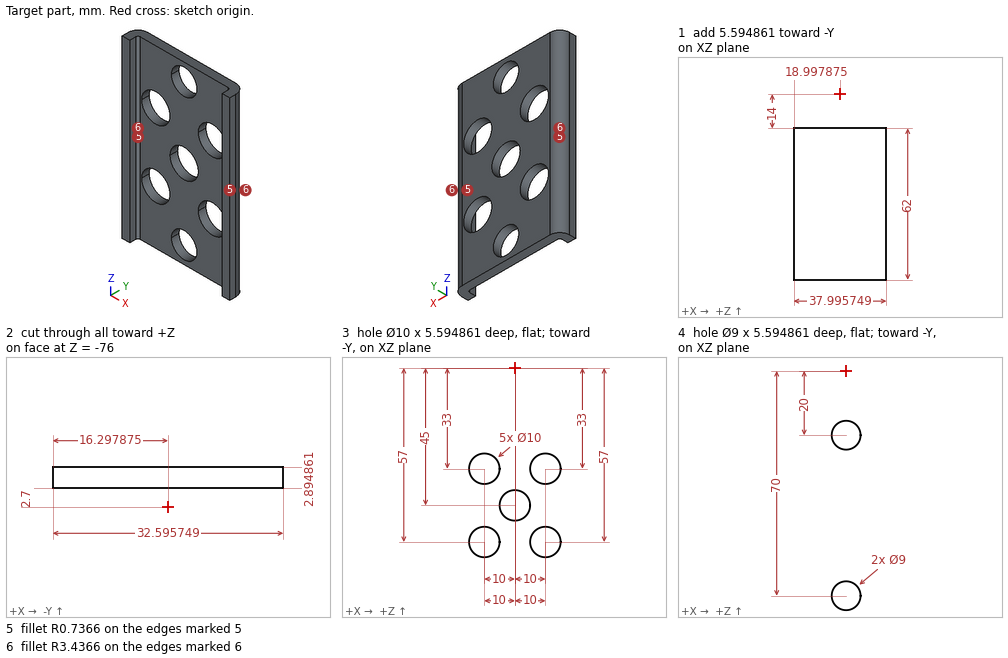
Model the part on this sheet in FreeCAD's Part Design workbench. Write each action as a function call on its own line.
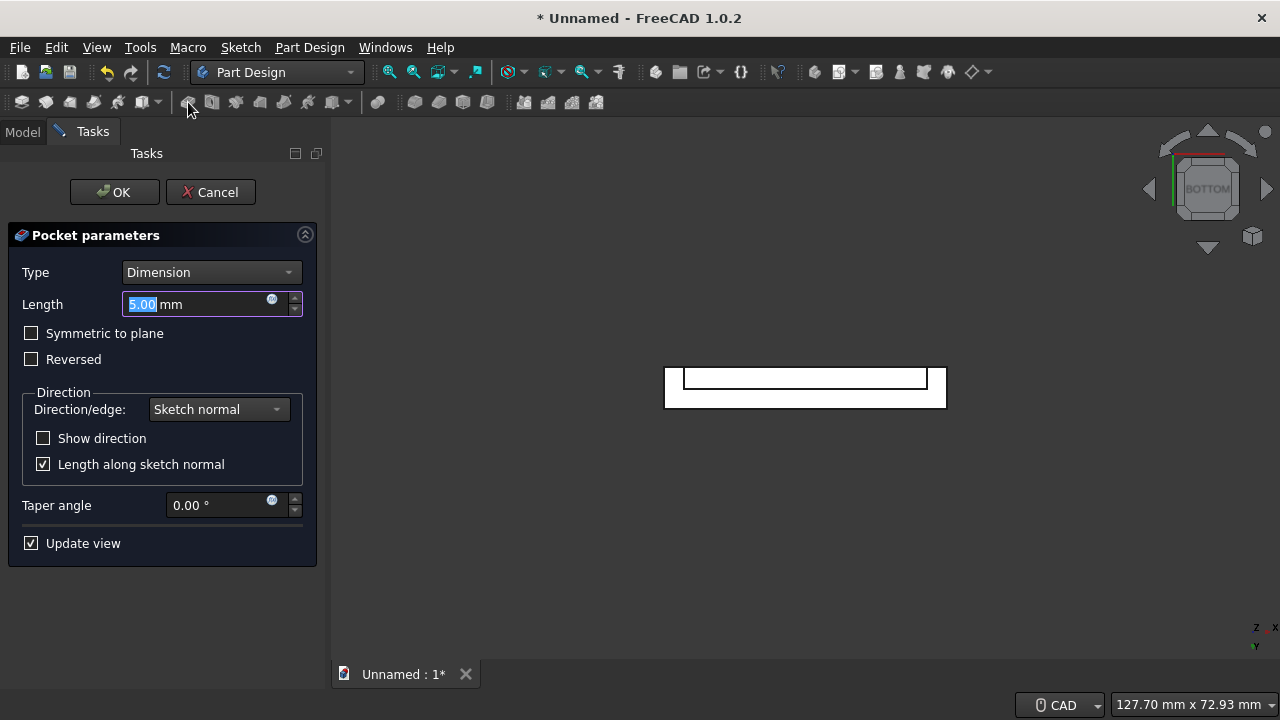
click(212, 272)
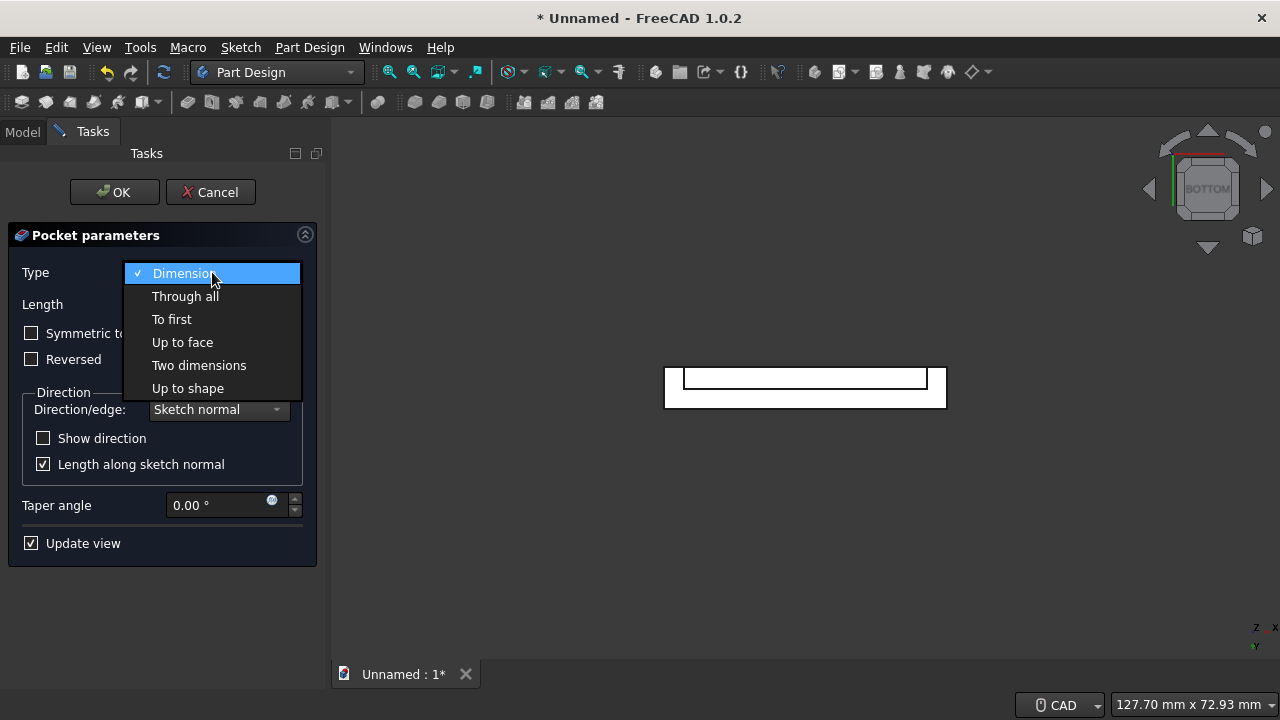
click(212, 296)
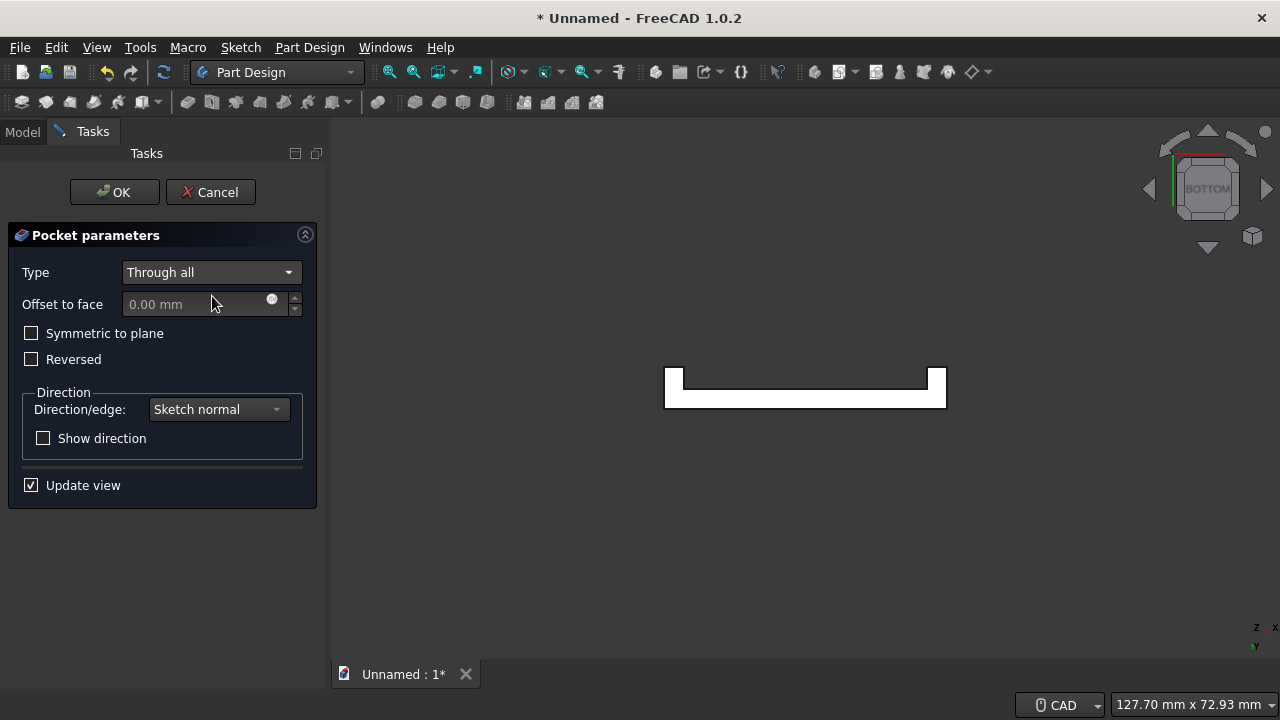
click(115, 192)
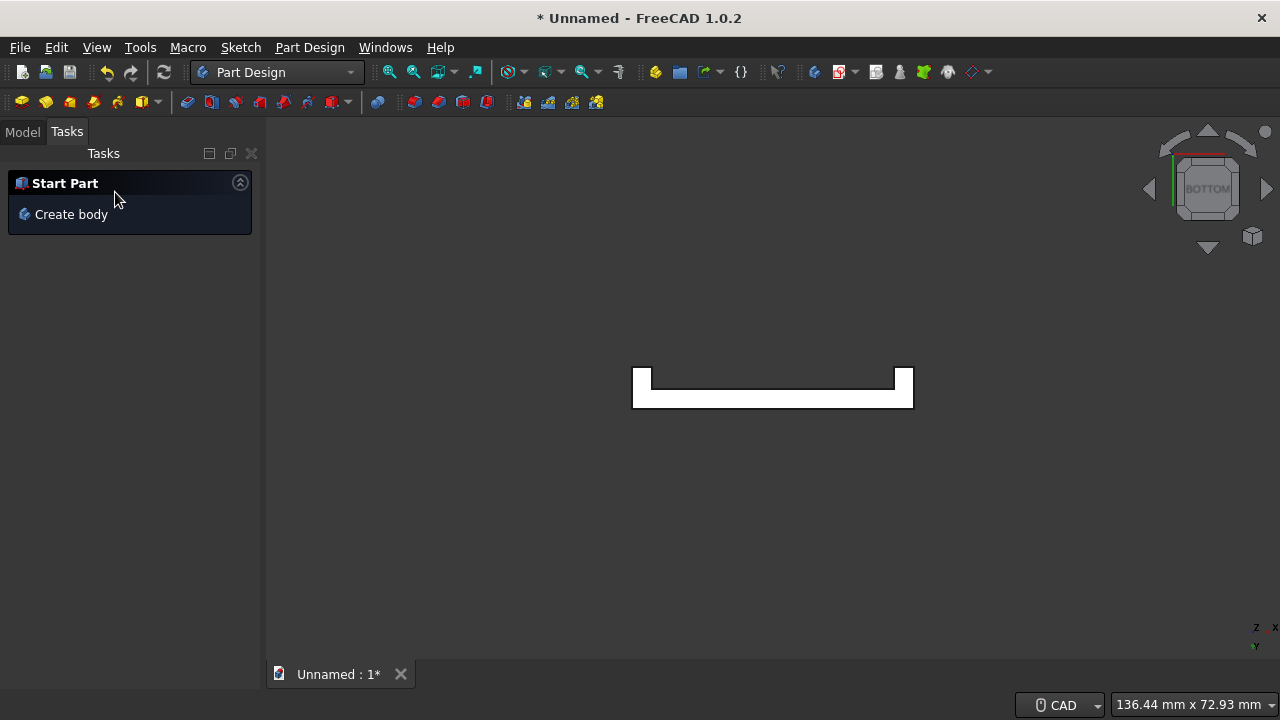
key(v)
key(f)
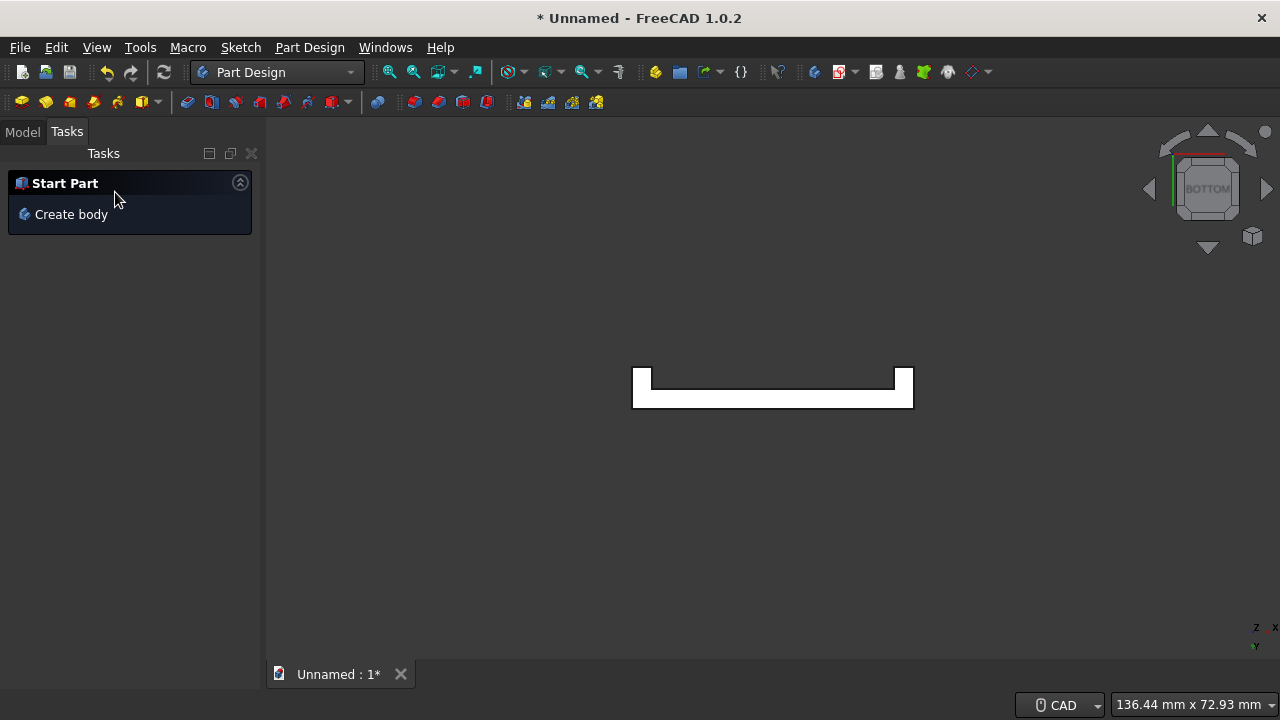
click(840, 72)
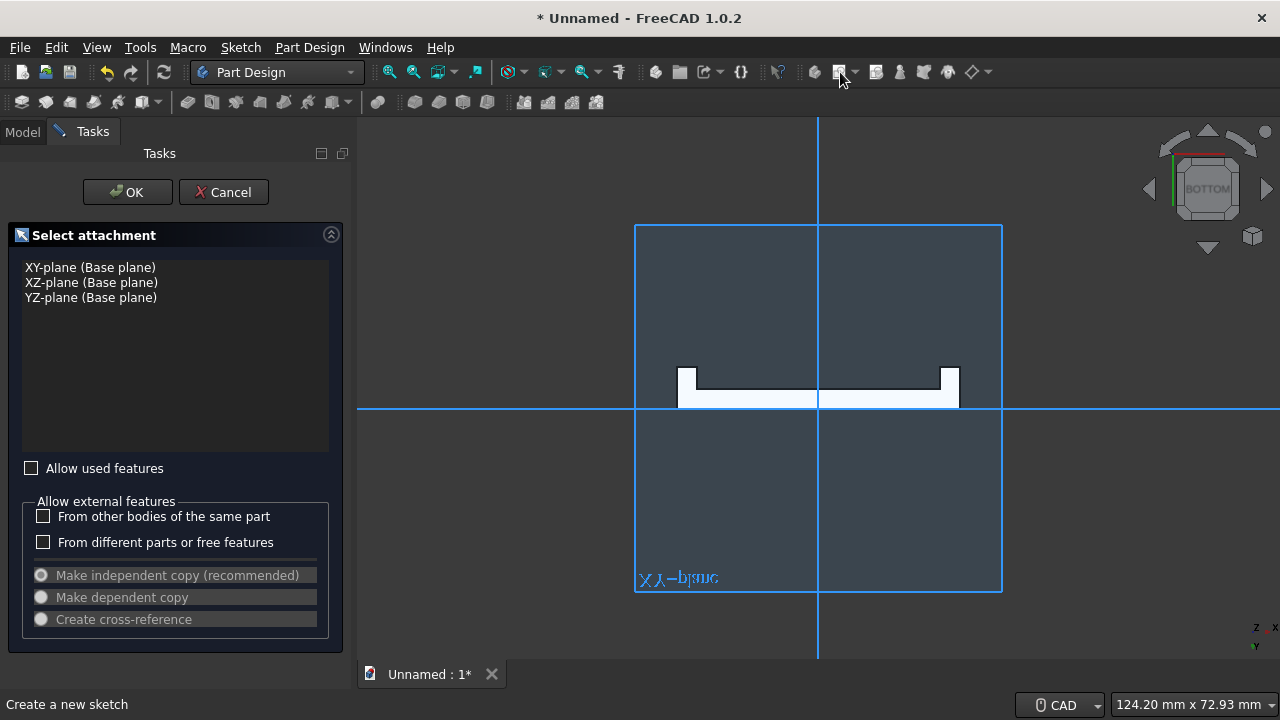
click(82, 282)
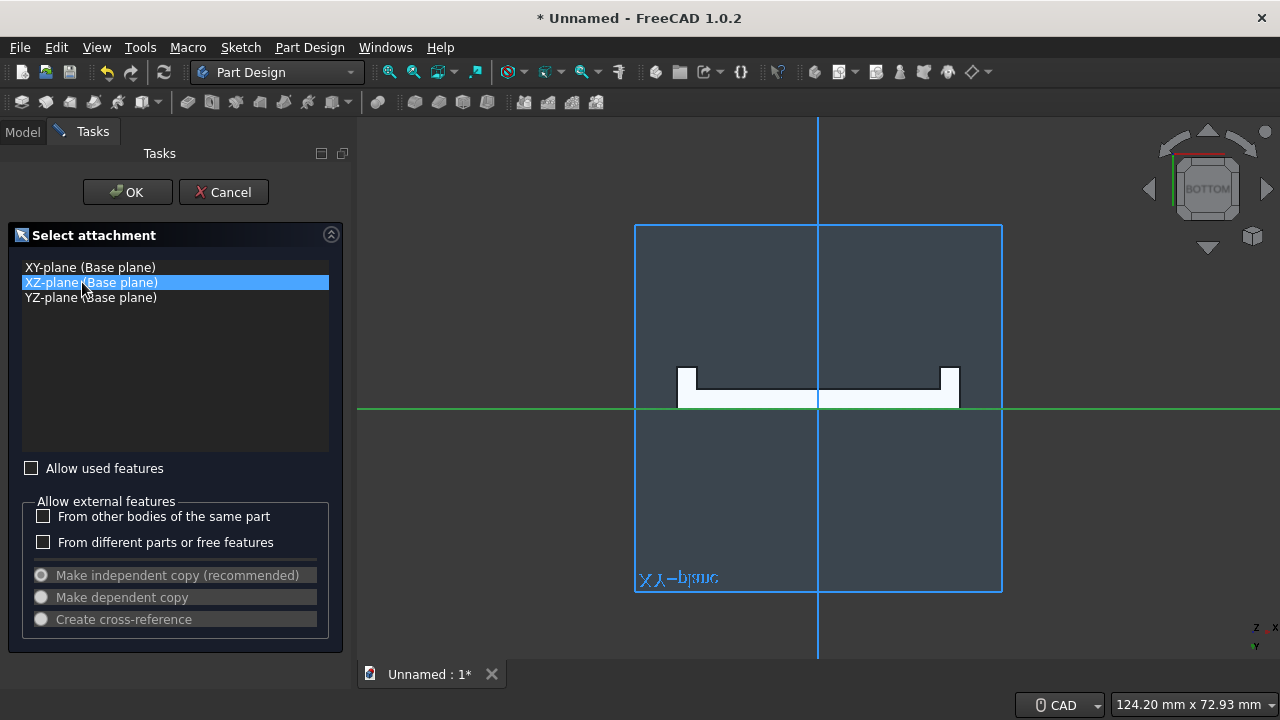
click(128, 192)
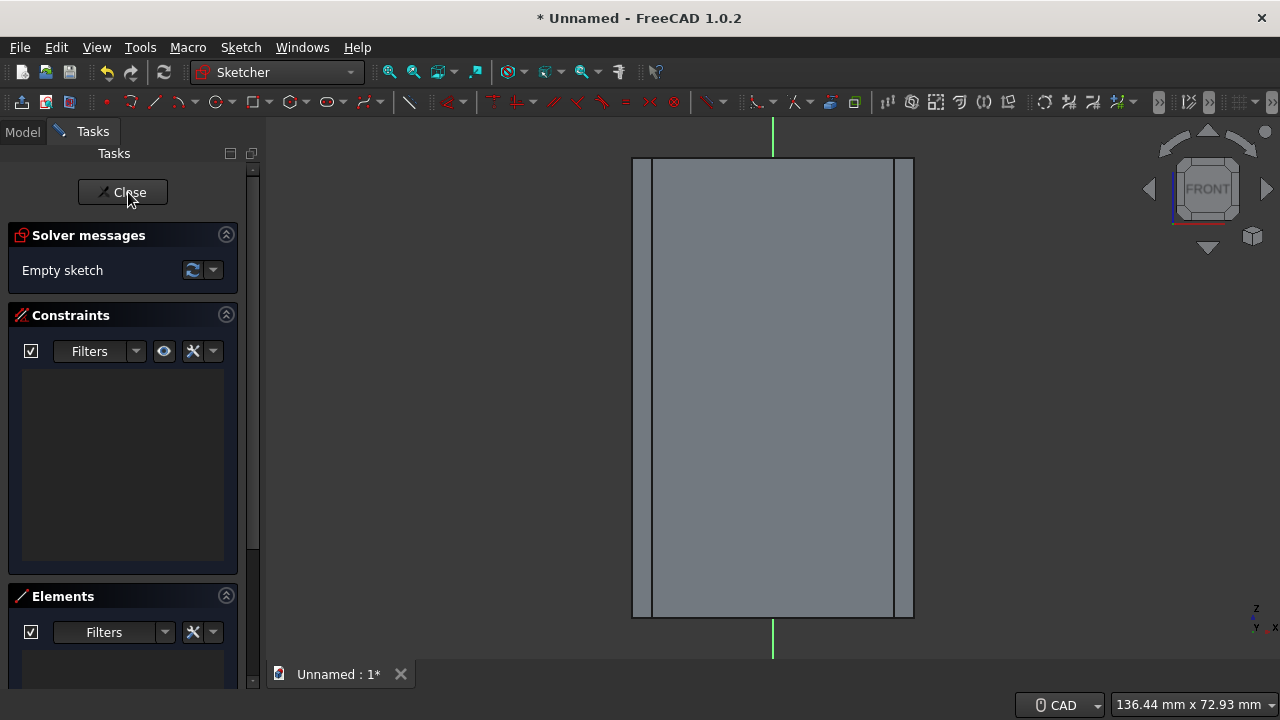
key(q)
key(s)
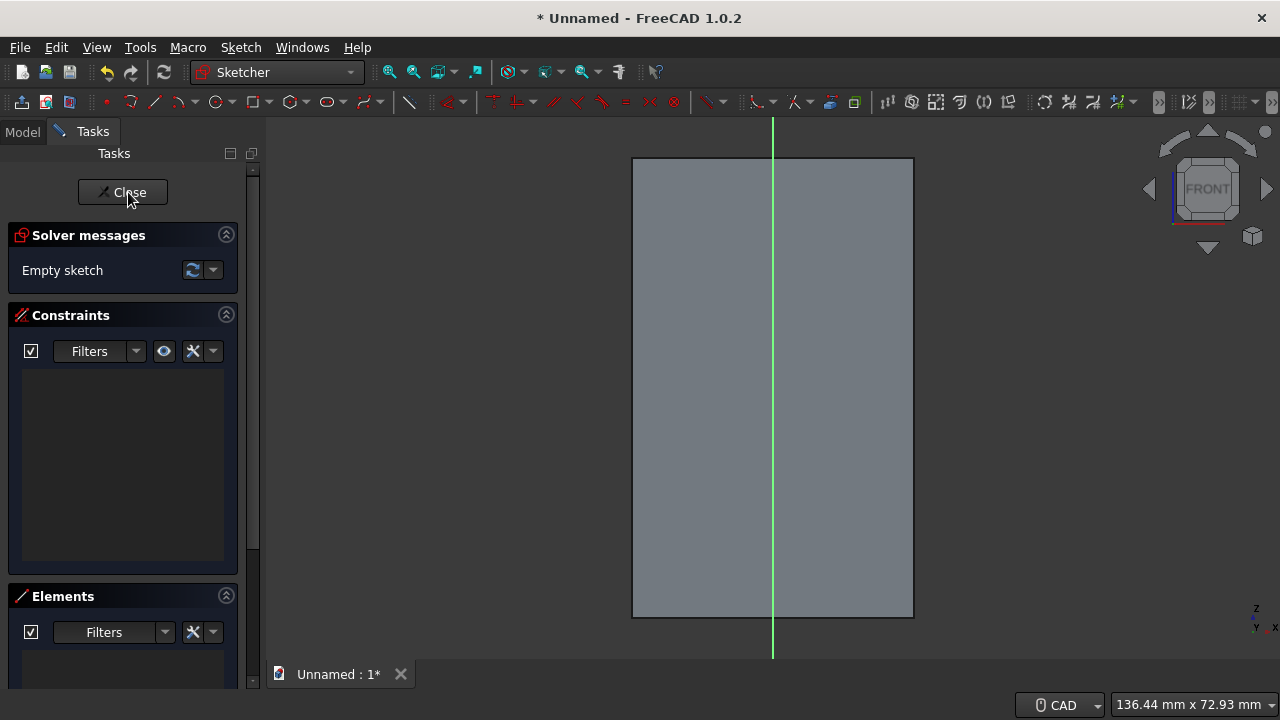
scroll(565, 600, down, 2)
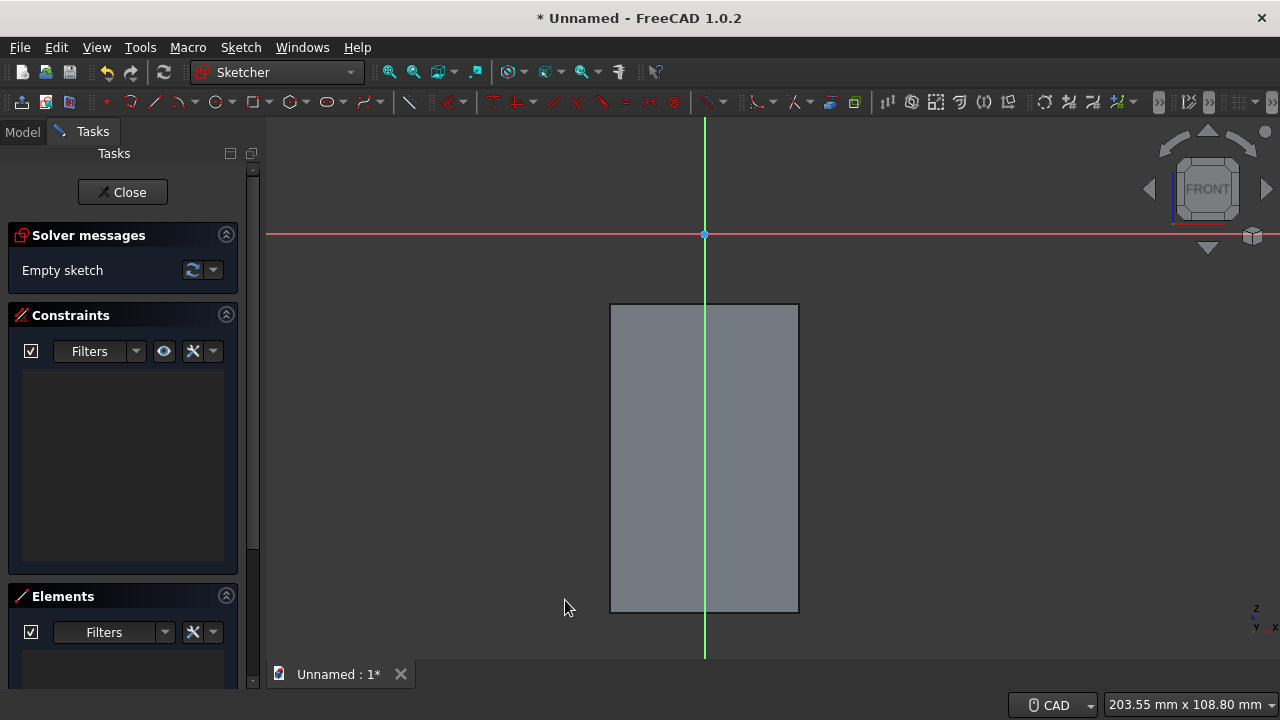
key(g)
key(c)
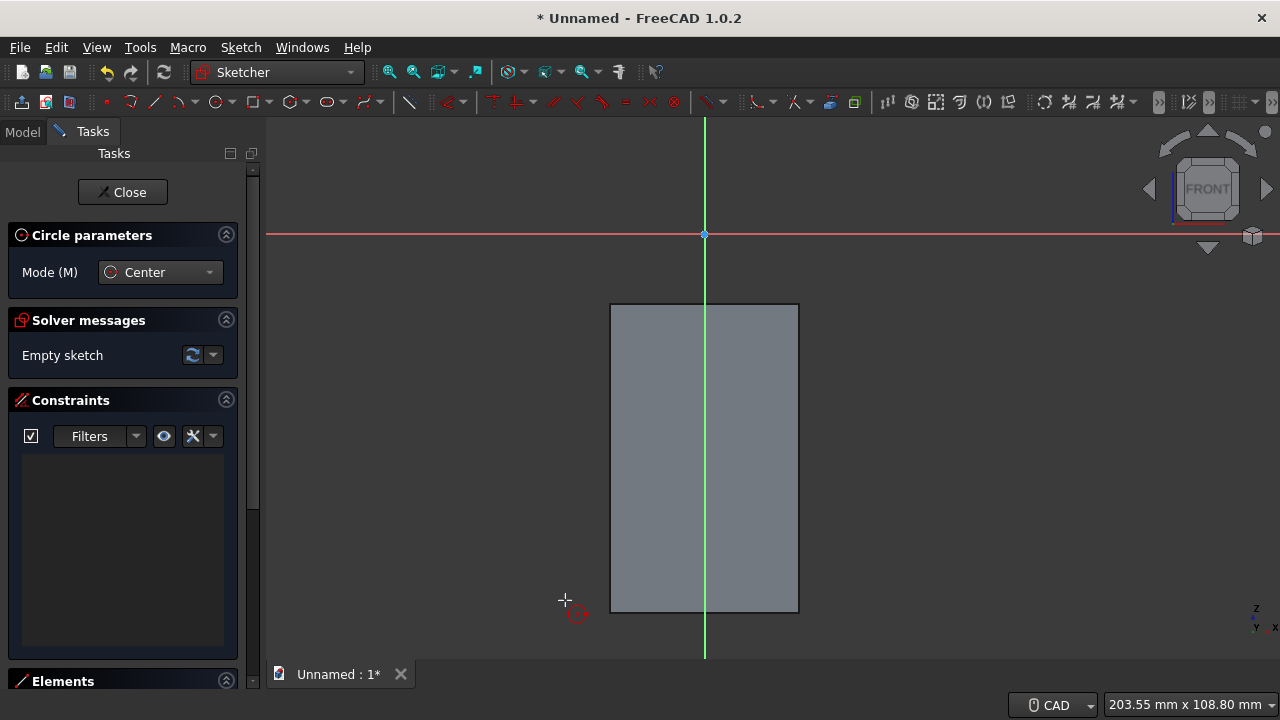
click(705, 458)
move(722, 441)